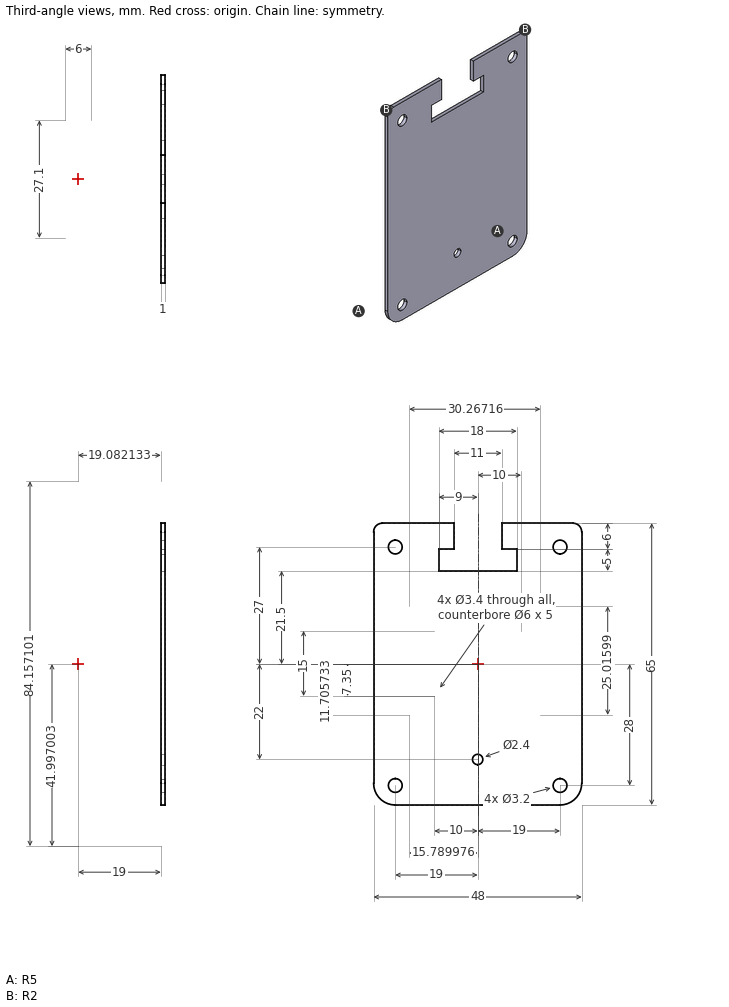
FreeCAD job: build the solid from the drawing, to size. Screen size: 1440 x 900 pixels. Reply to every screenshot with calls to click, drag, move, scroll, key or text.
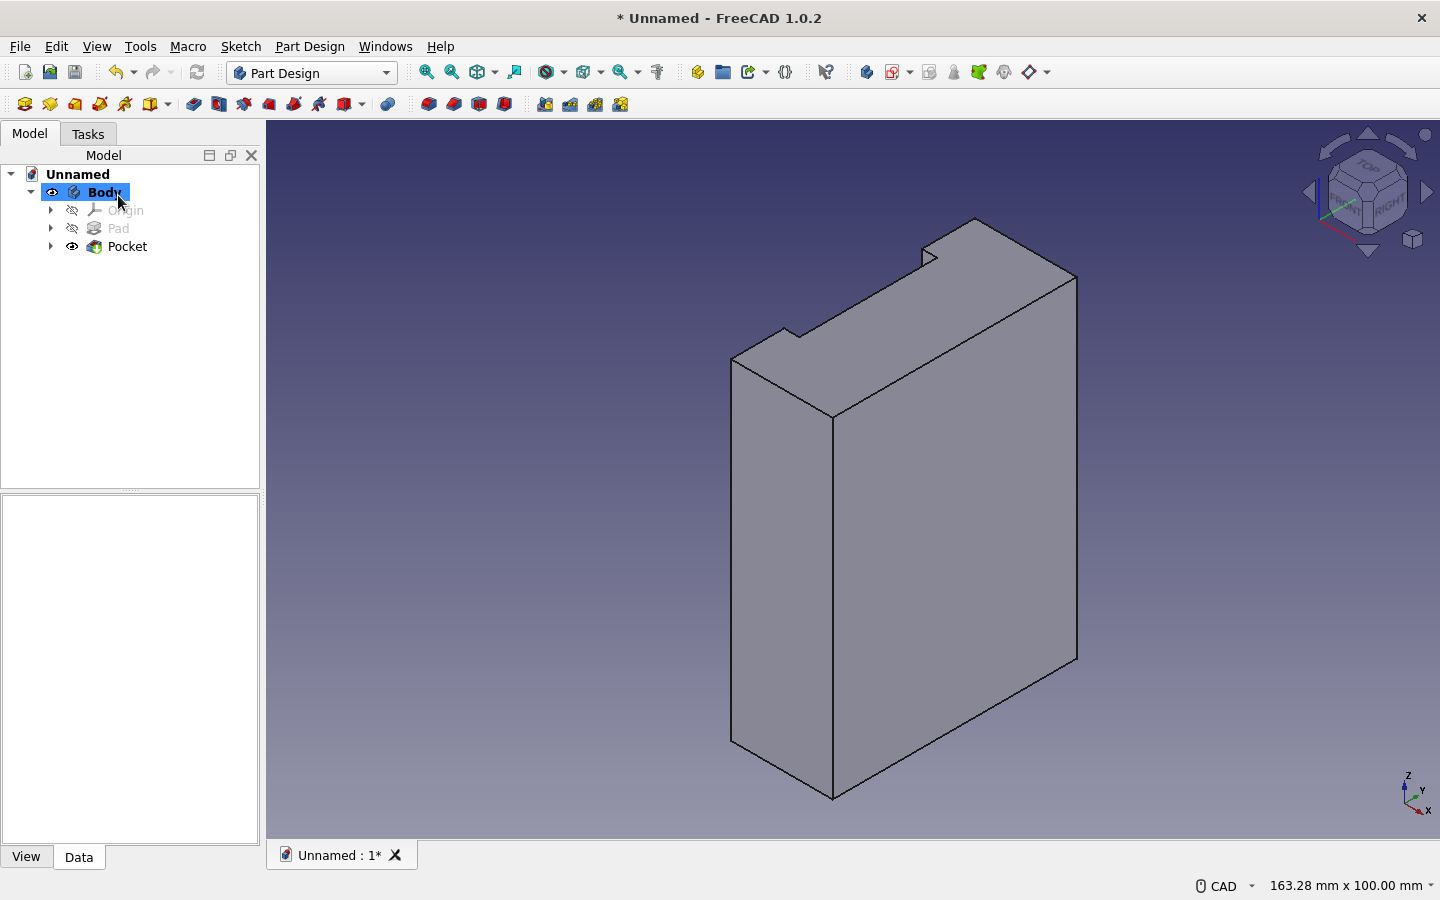
click(955, 537)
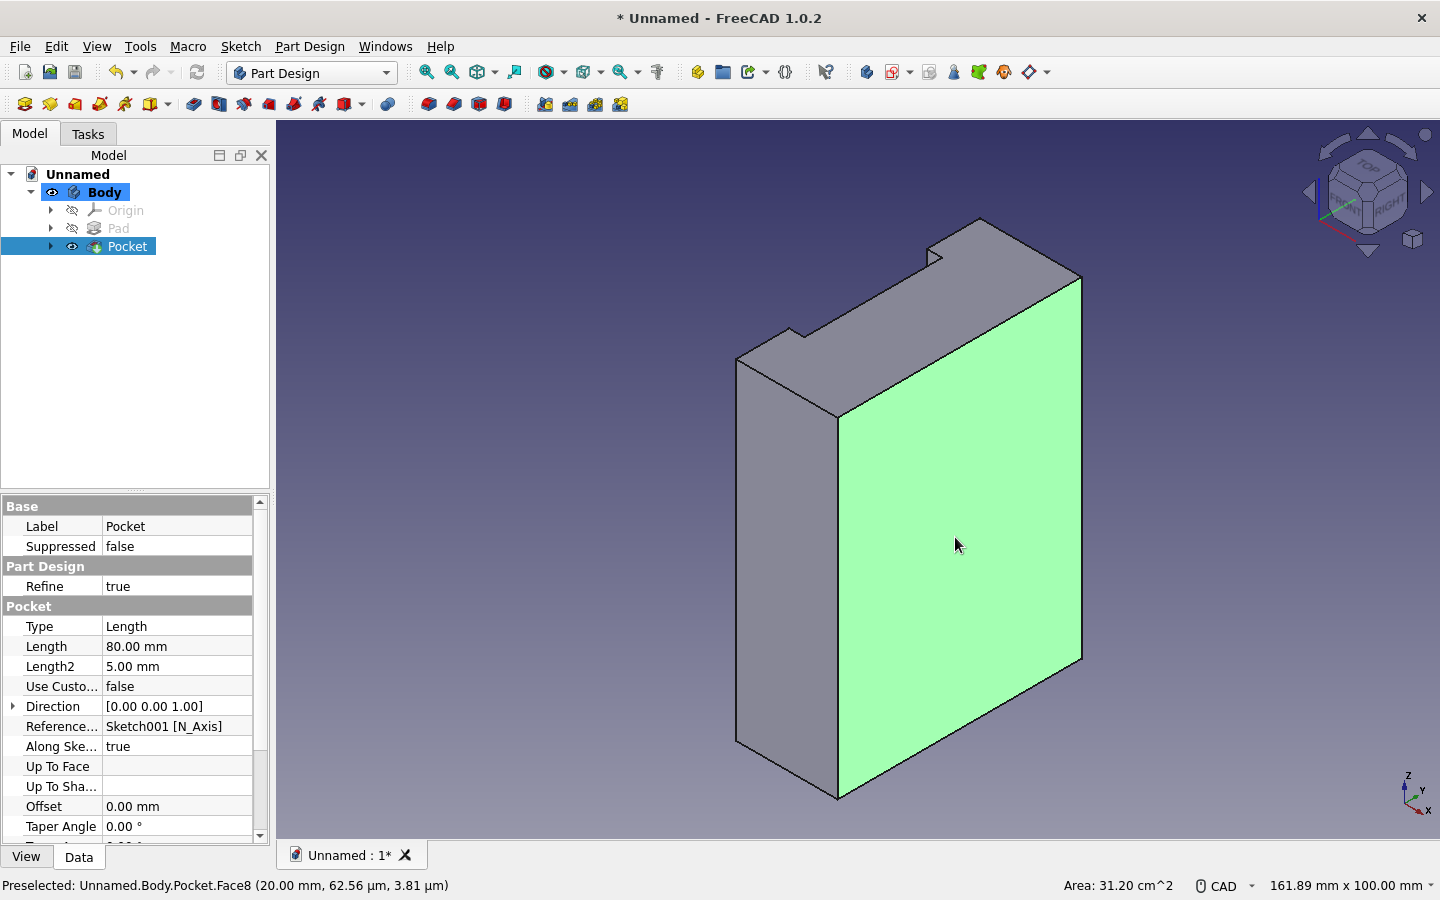
click(892, 72)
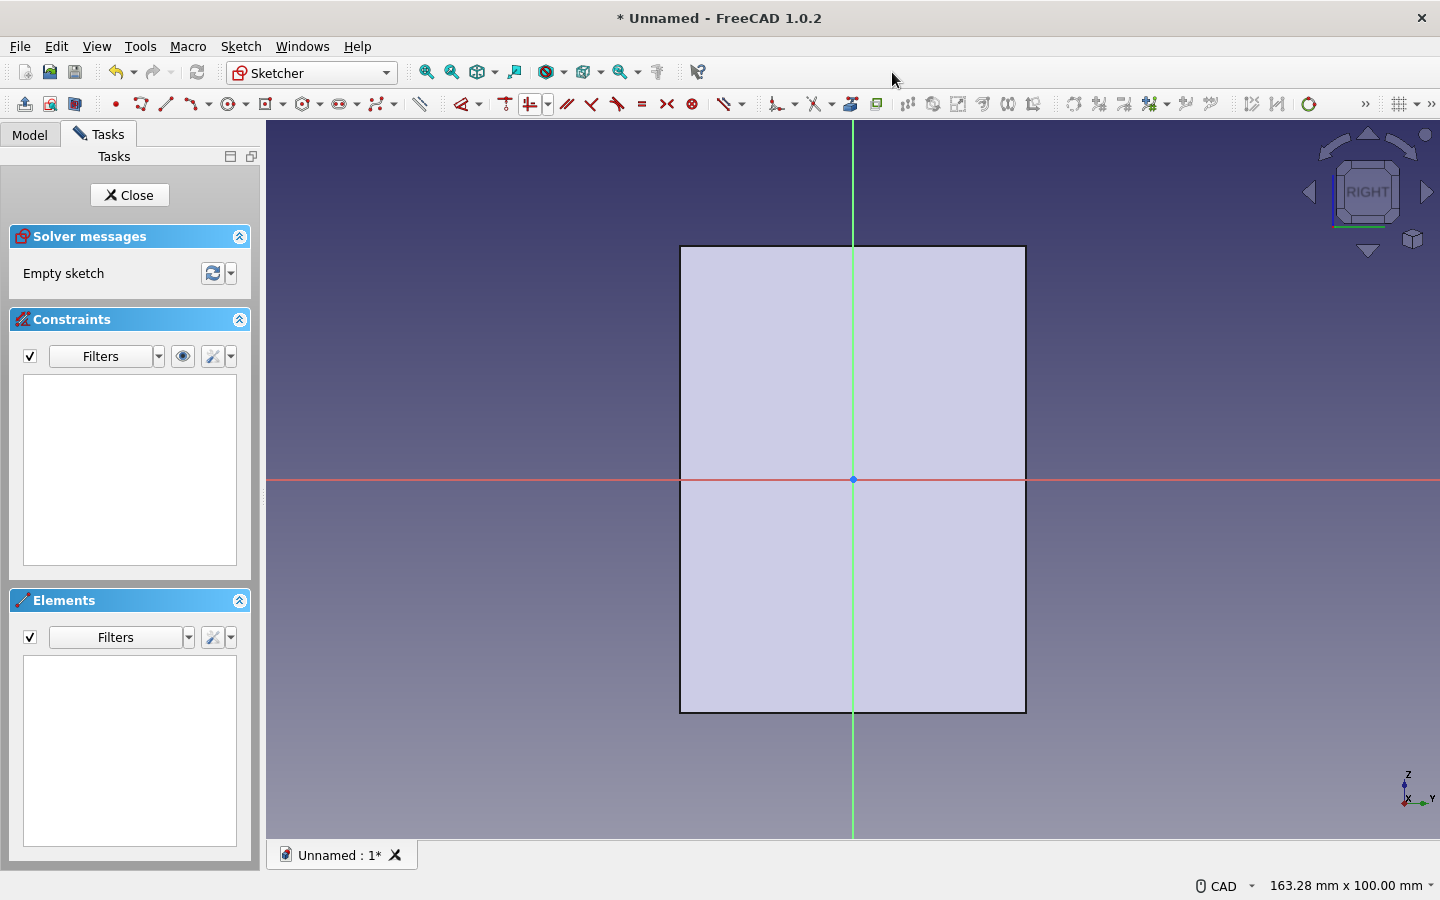
scroll(936, 221, up, 3)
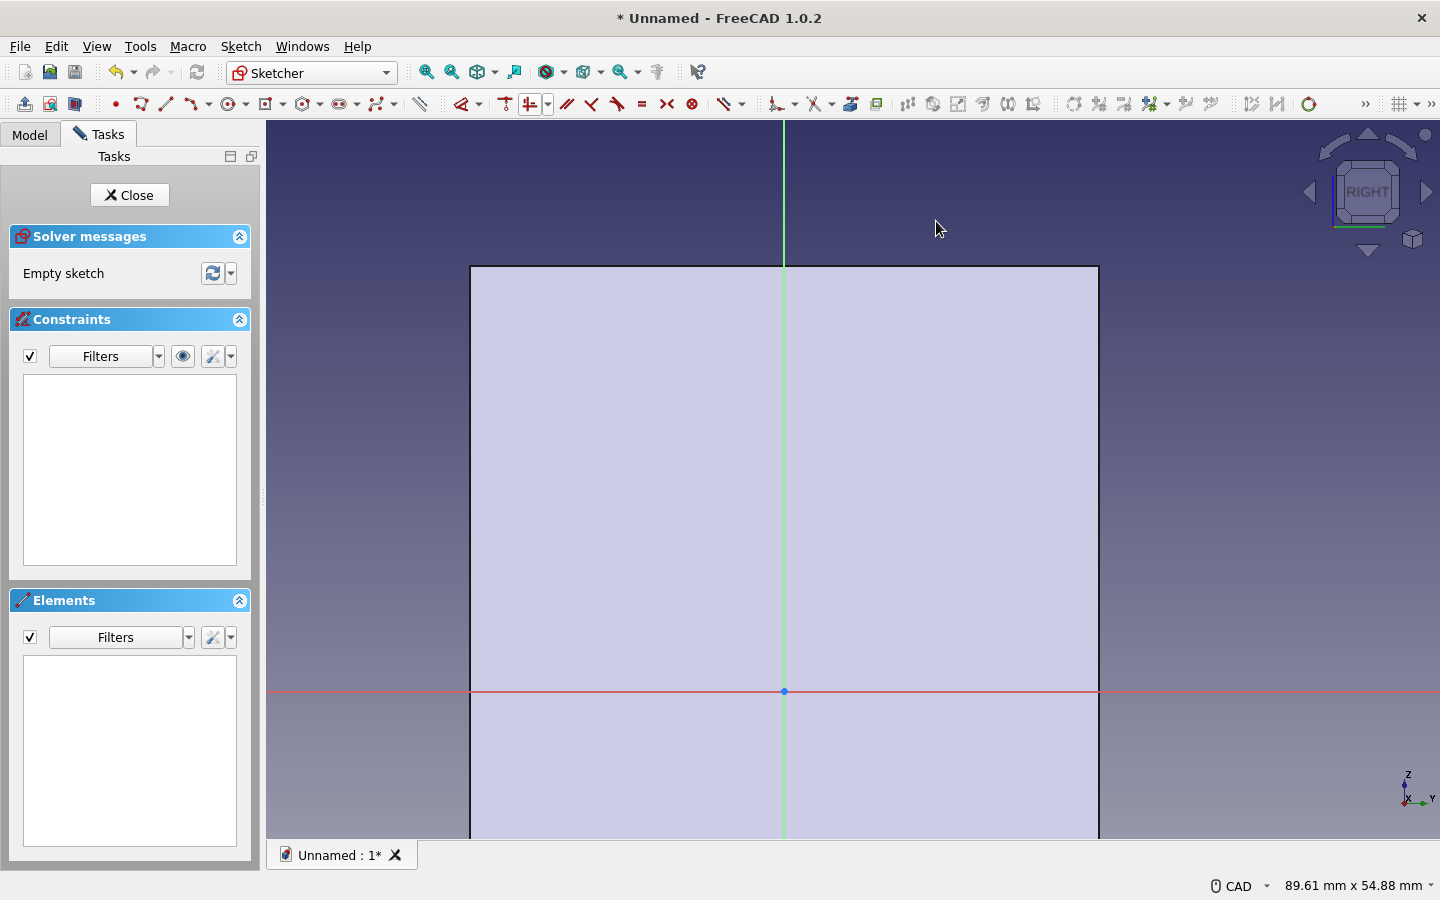
key(g)
key(m)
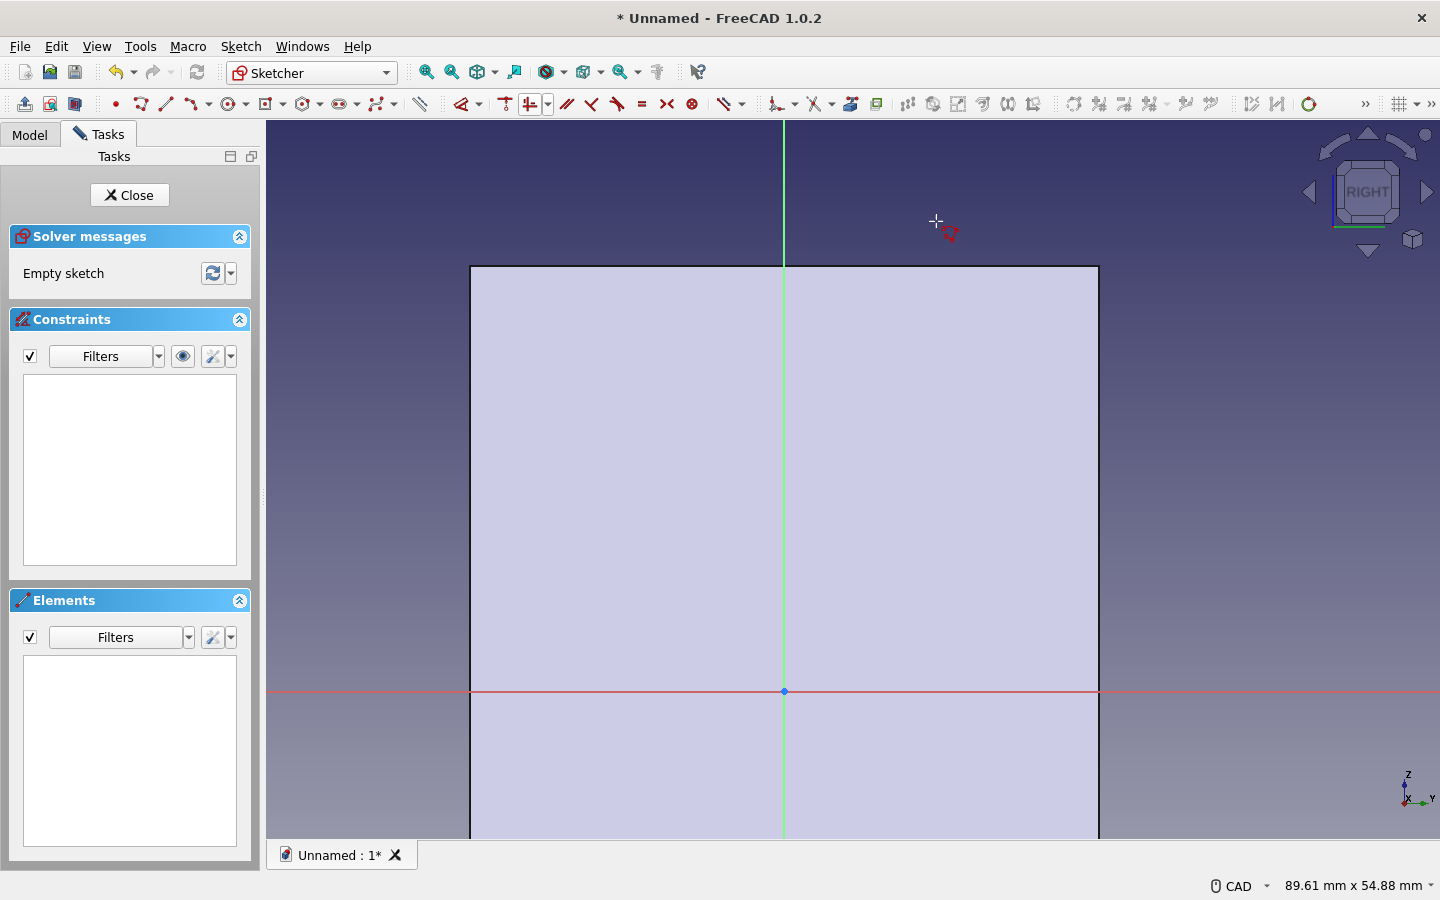
click(666, 410)
click(902, 410)
click(902, 345)
click(856, 345)
click(856, 266)
click(712, 266)
click(712, 345)
click(666, 345)
click(666, 411)
key(Escape)
key(Escape)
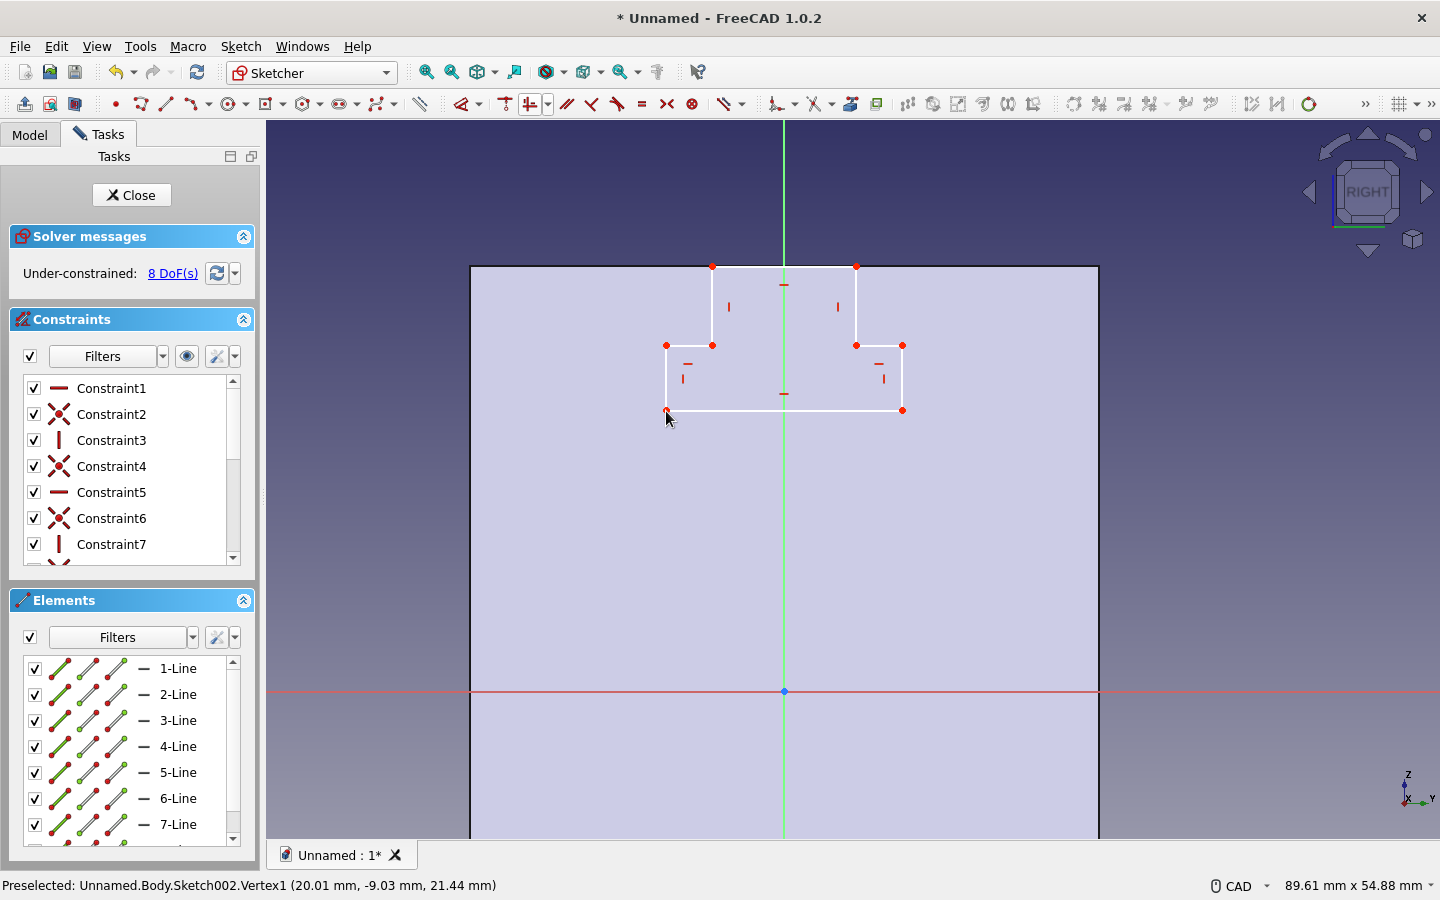
click(856, 346)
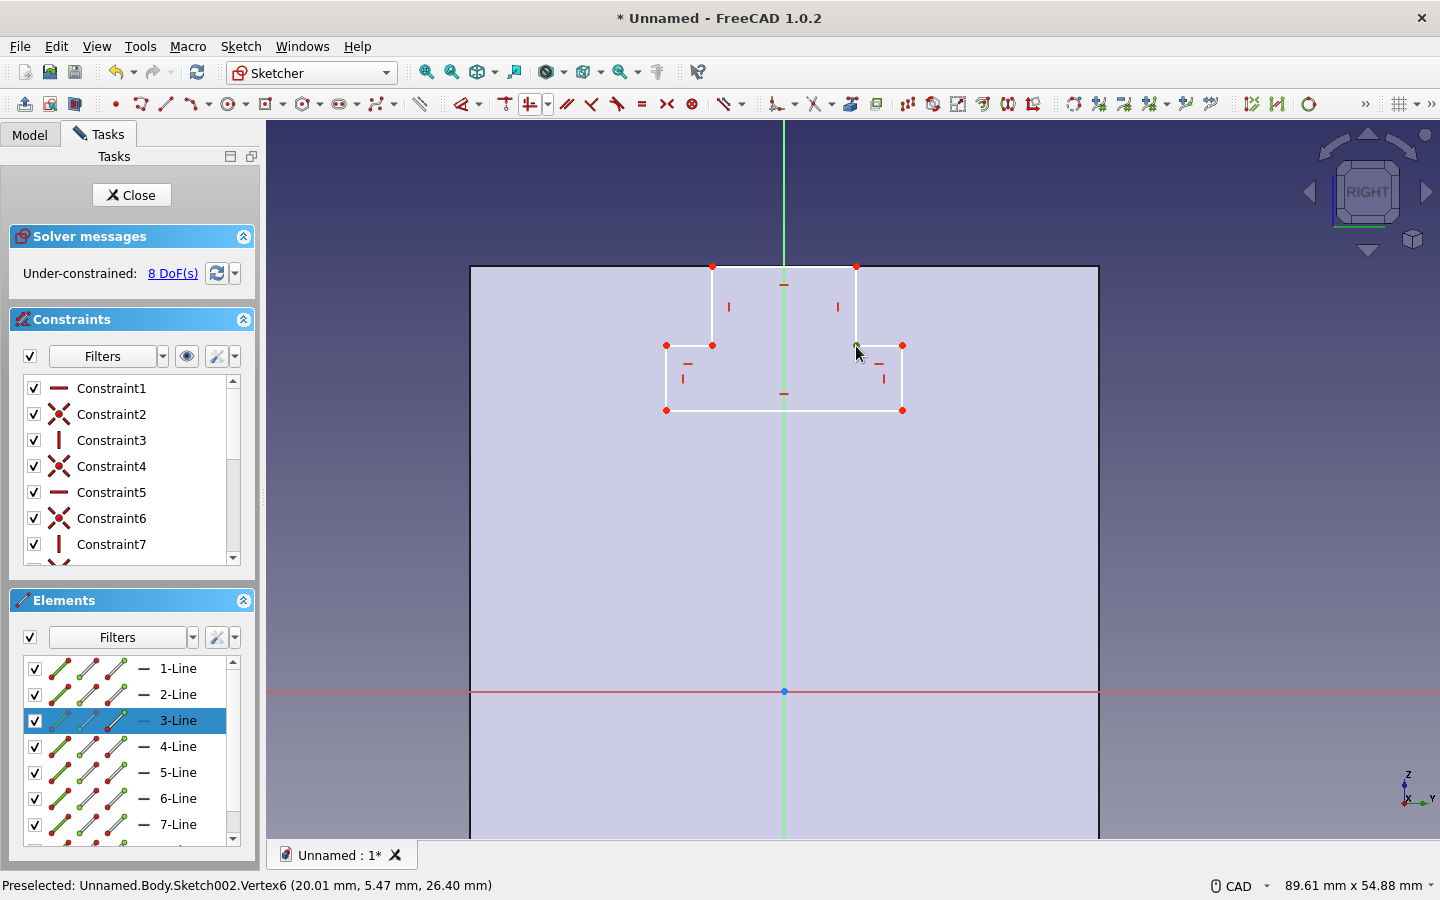
click(712, 346)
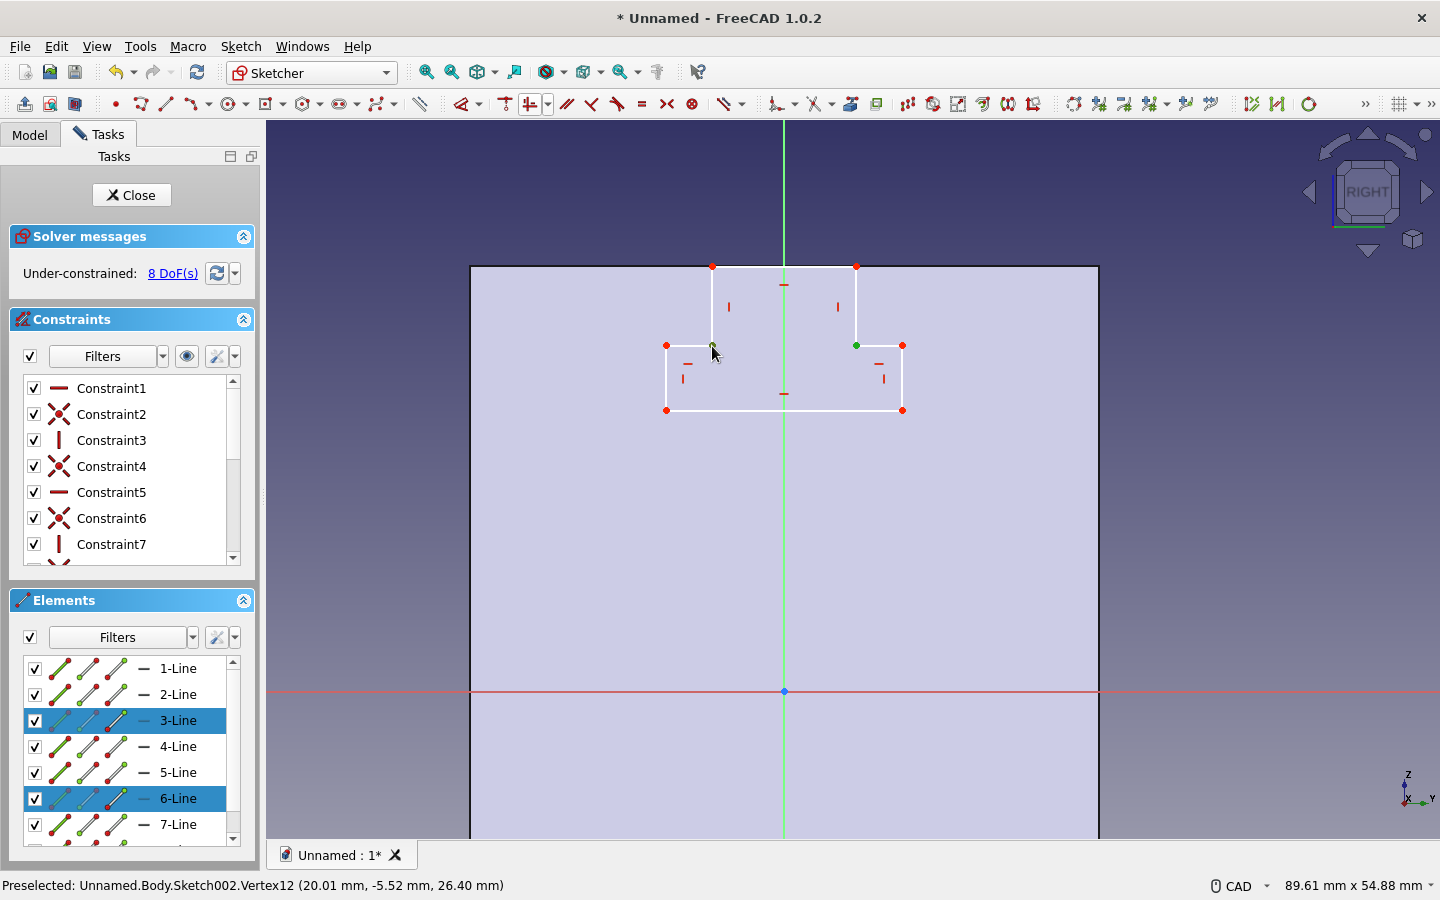
click(784, 764)